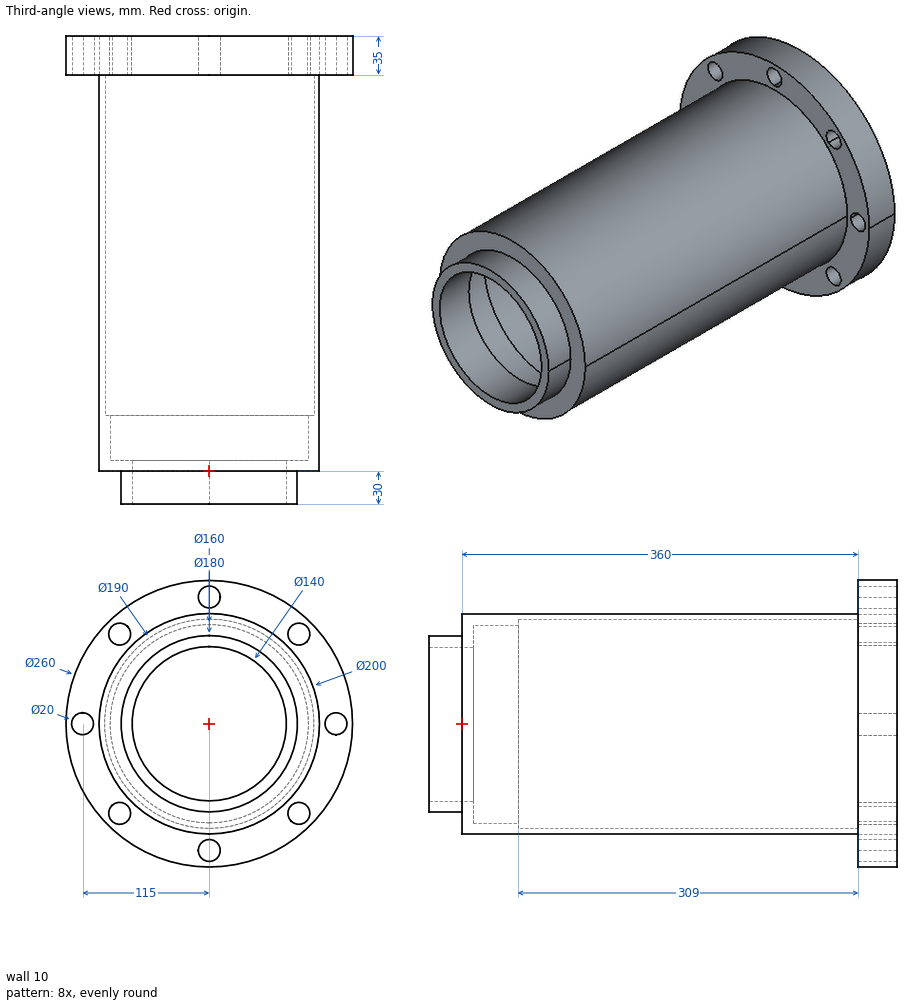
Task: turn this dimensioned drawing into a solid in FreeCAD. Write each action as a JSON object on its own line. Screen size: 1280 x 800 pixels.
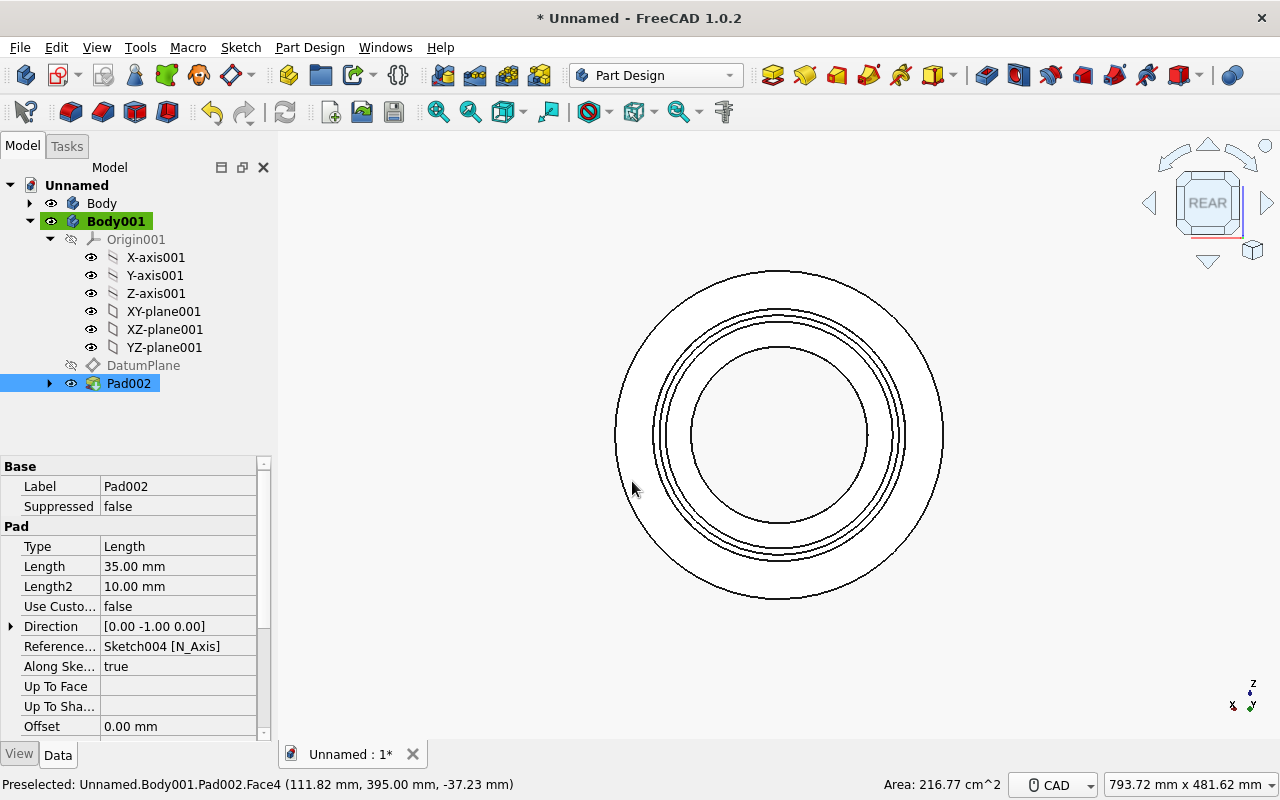
{"action": "left_click", "coordinate": [58, 76]}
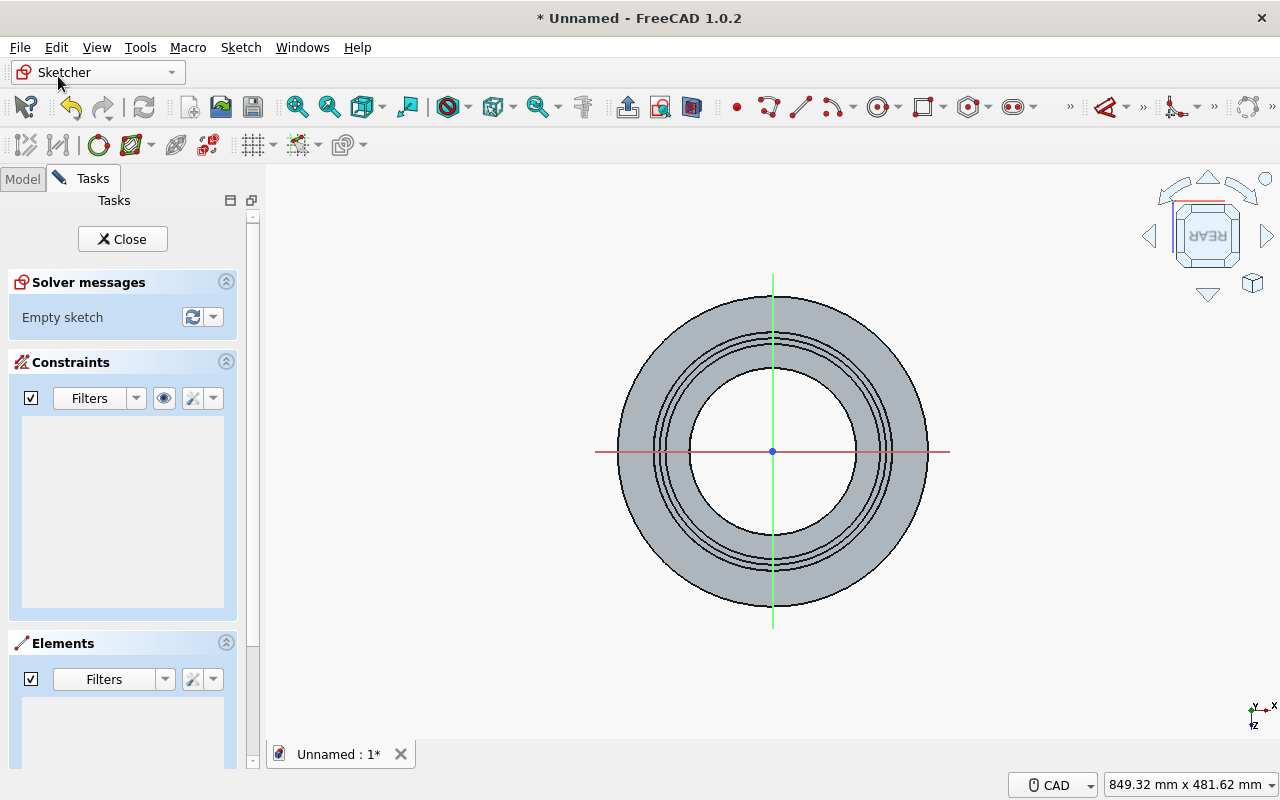
{"action": "scroll", "coordinate": [631, 451], "scroll_direction": "up", "scroll_amount": 14}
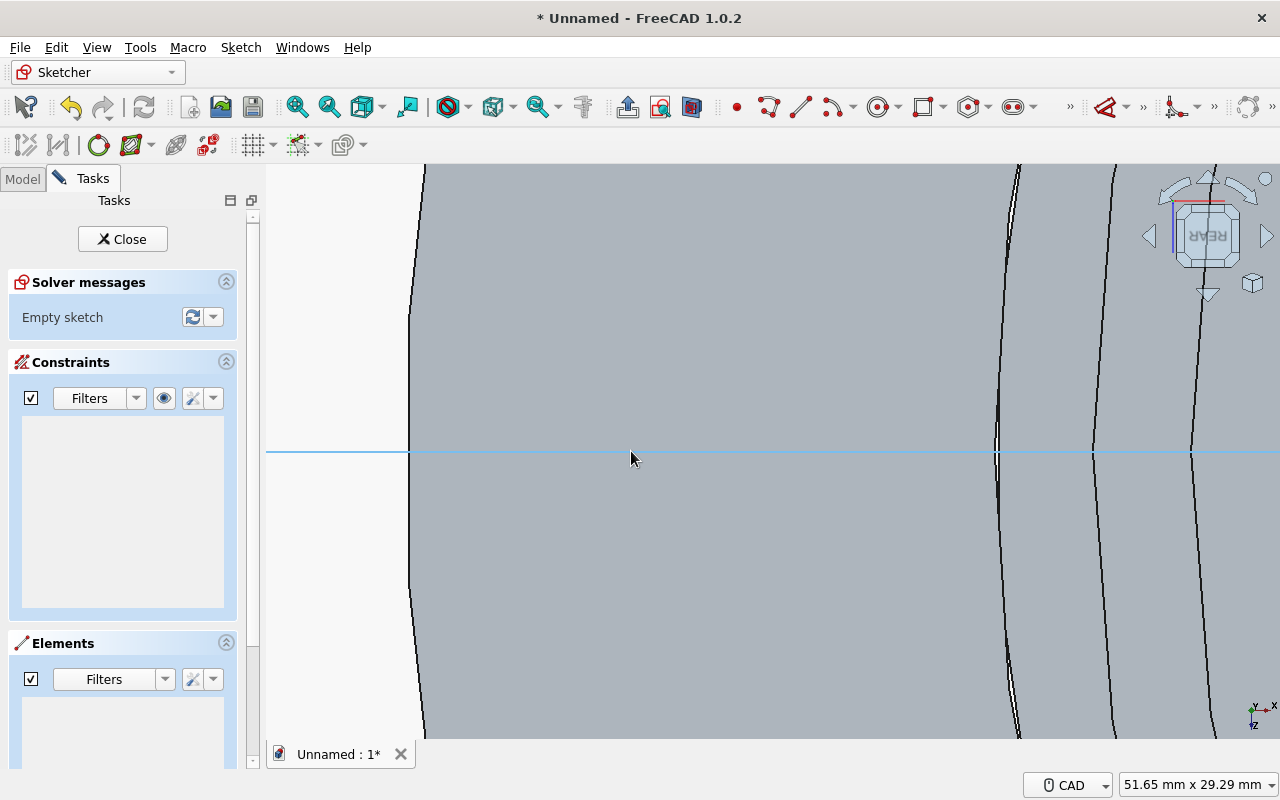
{"action": "key", "text": "g c"}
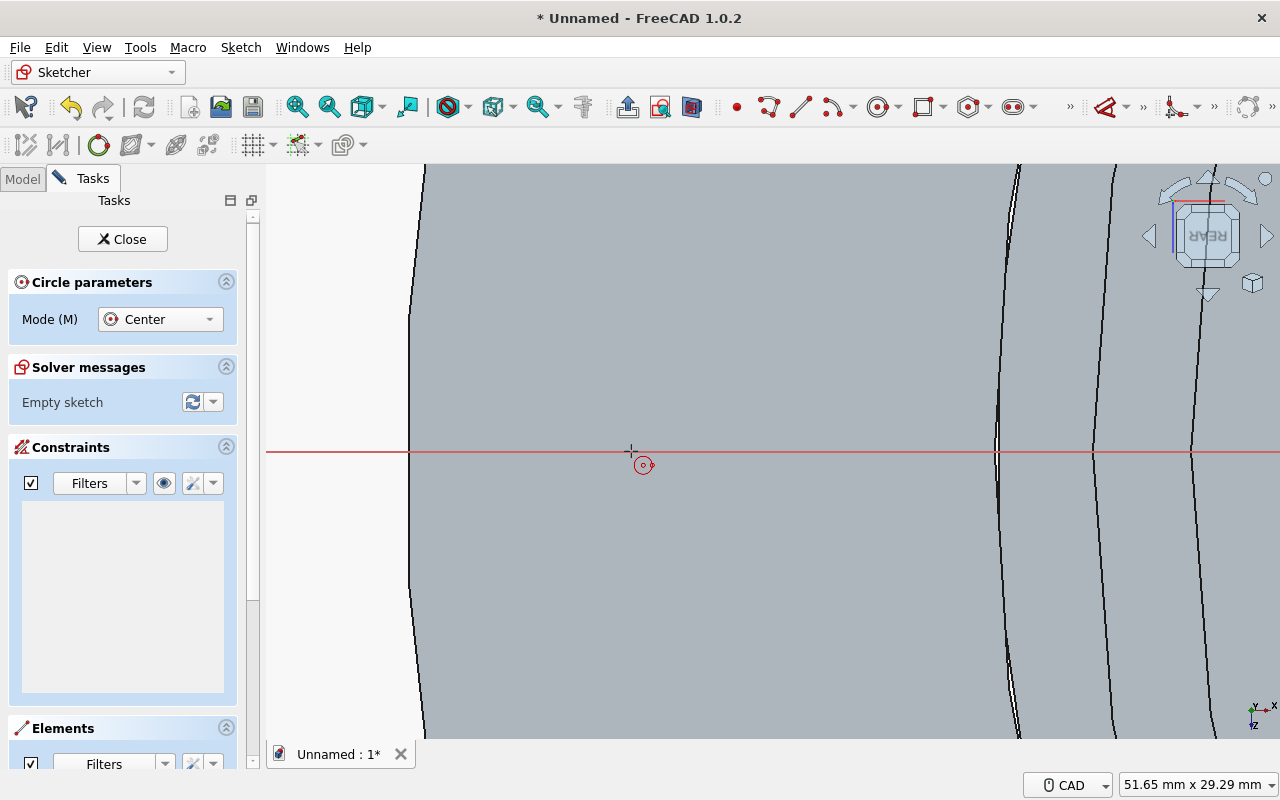
{"action": "left_click", "coordinate": [700, 451]}
{"action": "left_click", "coordinate": [839, 313]}
{"action": "key", "text": "Escape"}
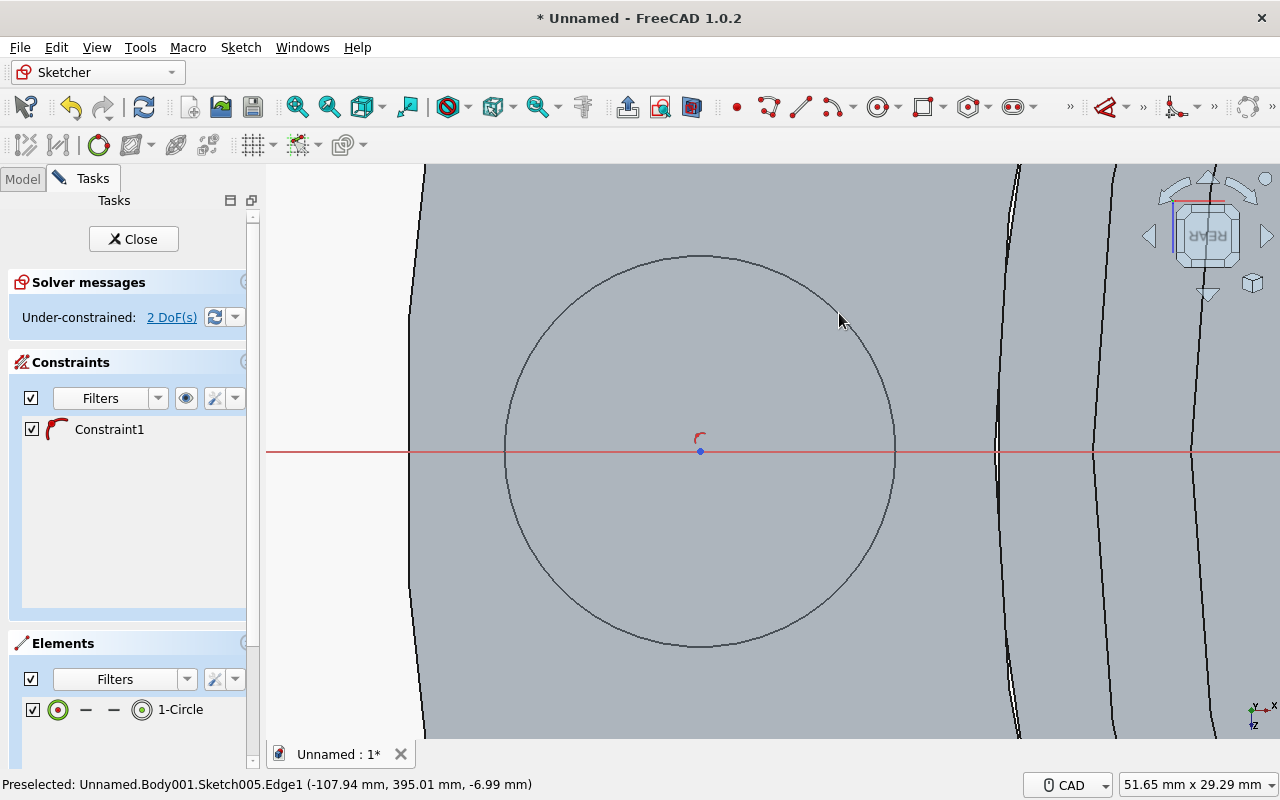
{"action": "left_click", "coordinate": [1106, 108]}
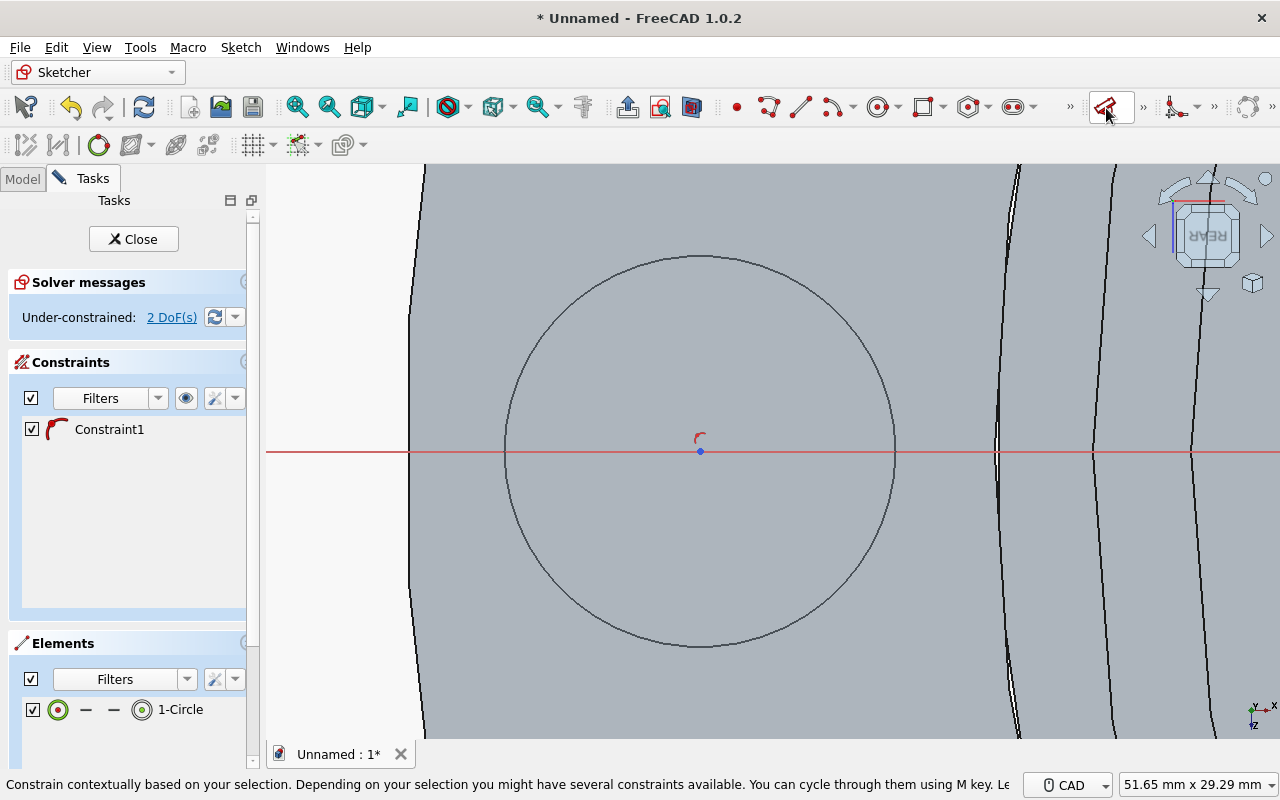
{"action": "left_click", "coordinate": [838, 313]}
{"action": "left_click", "coordinate": [861, 290]}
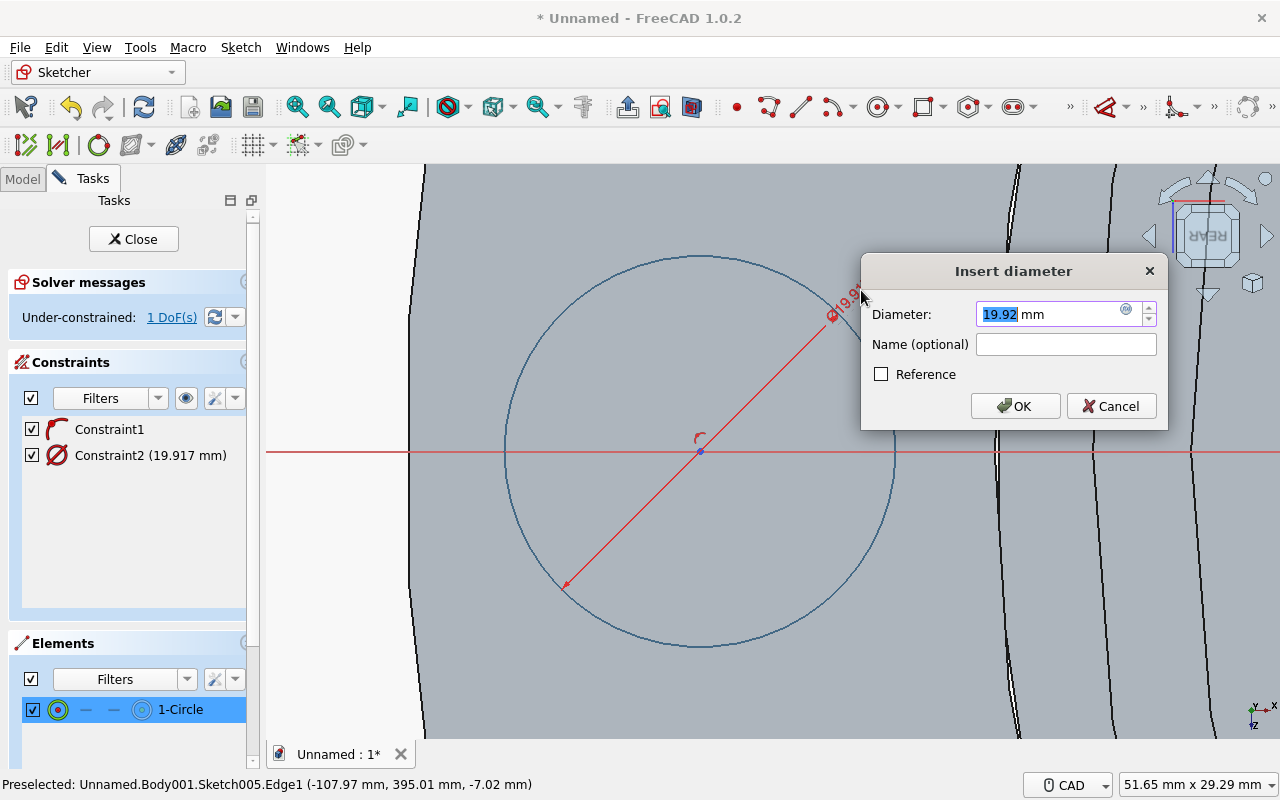
{"action": "type", "text": "20"}
{"action": "key", "text": "Return"}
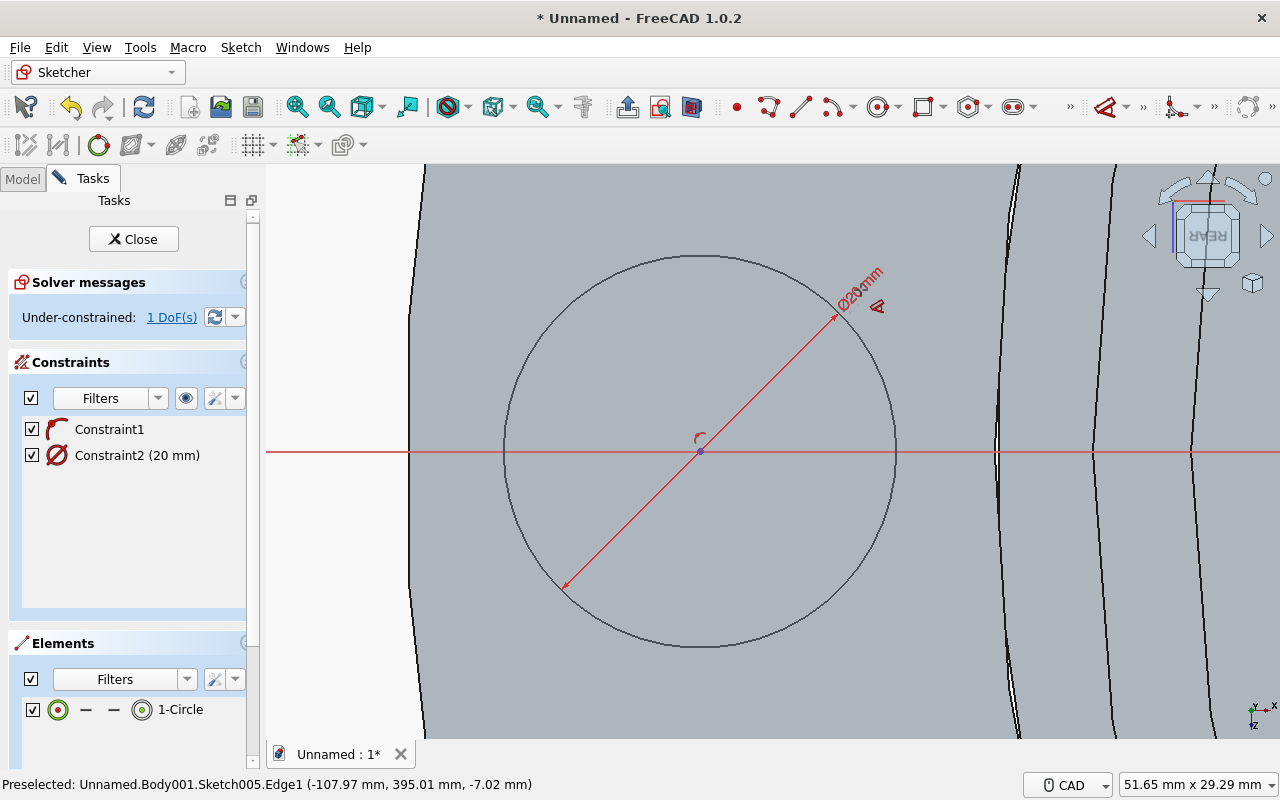
{"action": "left_click", "coordinate": [700, 451]}
{"action": "left_click", "coordinate": [908, 485]}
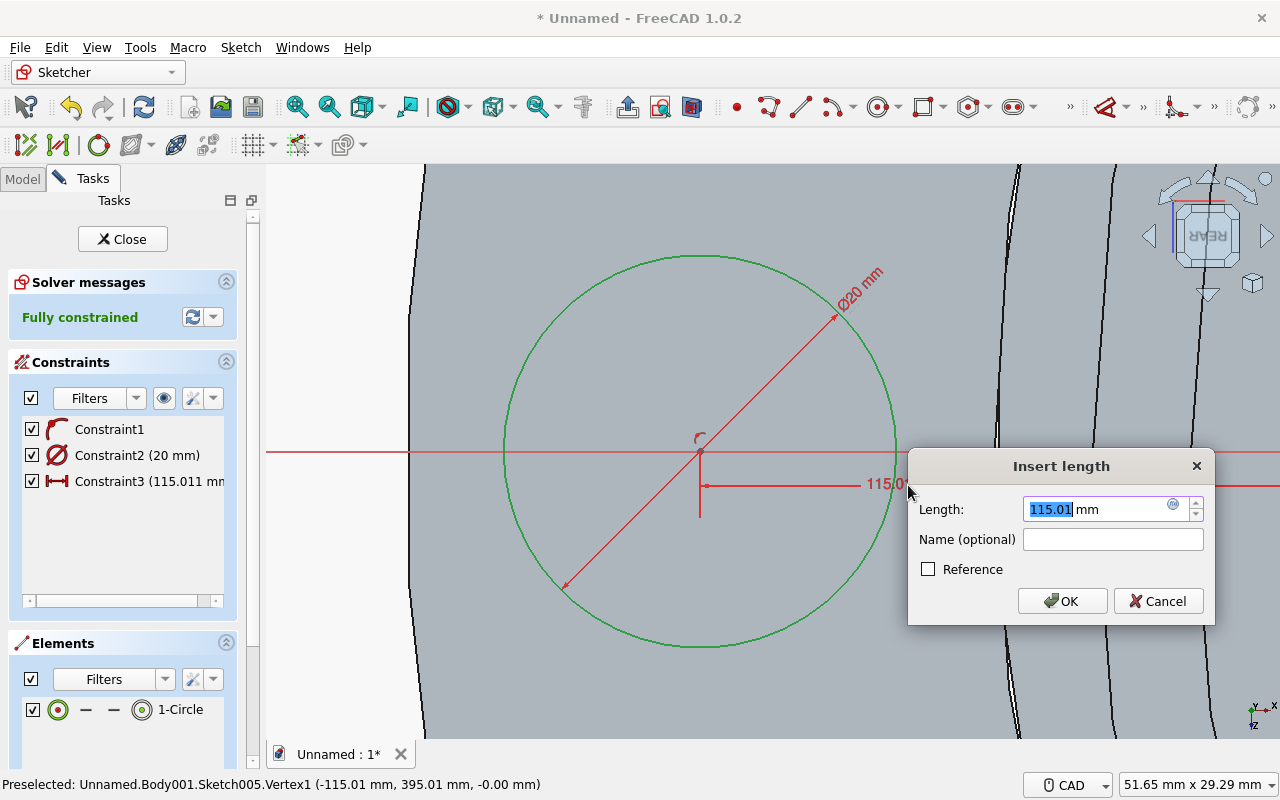
{"action": "type", "text": "115"}
{"action": "key", "text": "Return"}
{"action": "key", "text": "Escape"}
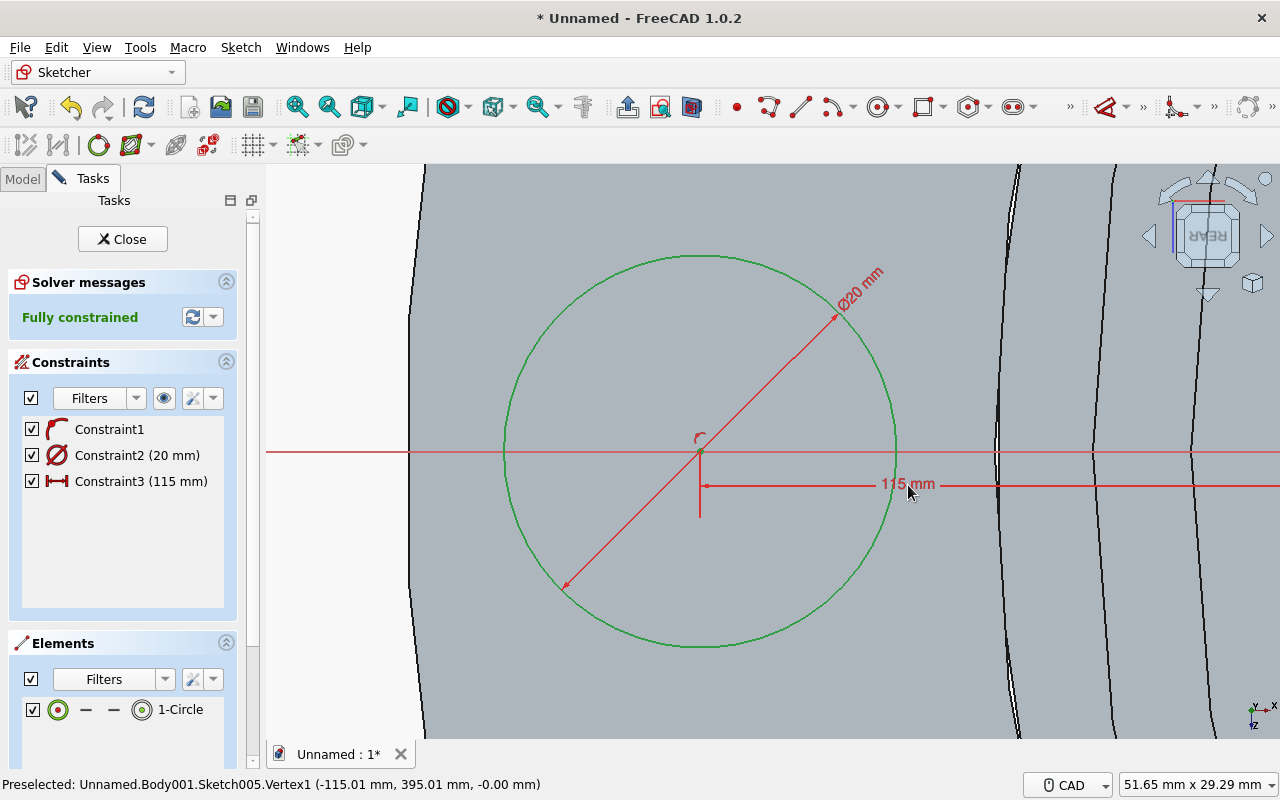
{"action": "left_click", "coordinate": [123, 239]}